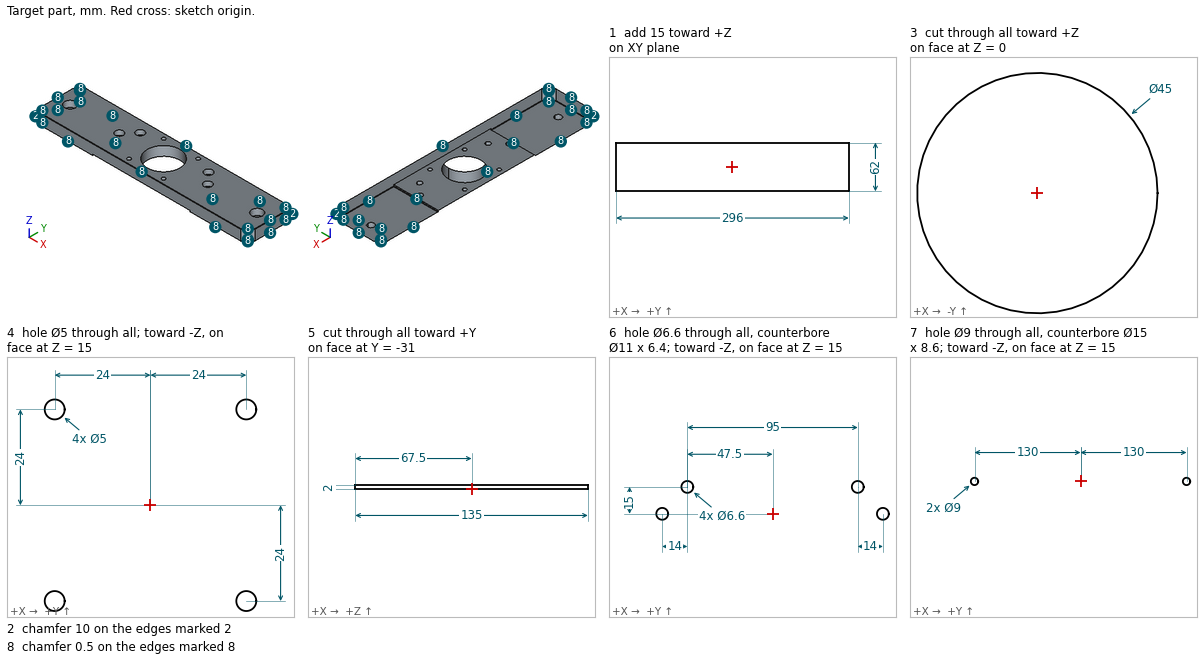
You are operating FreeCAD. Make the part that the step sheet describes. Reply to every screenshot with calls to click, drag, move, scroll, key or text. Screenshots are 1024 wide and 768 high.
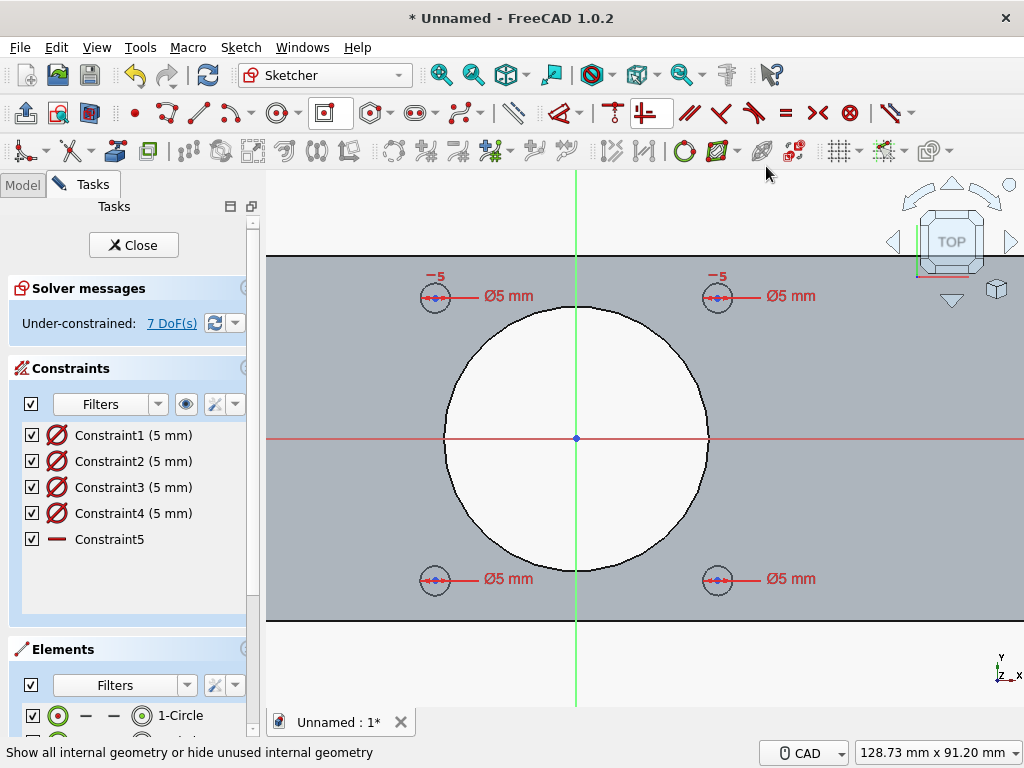
click(718, 298)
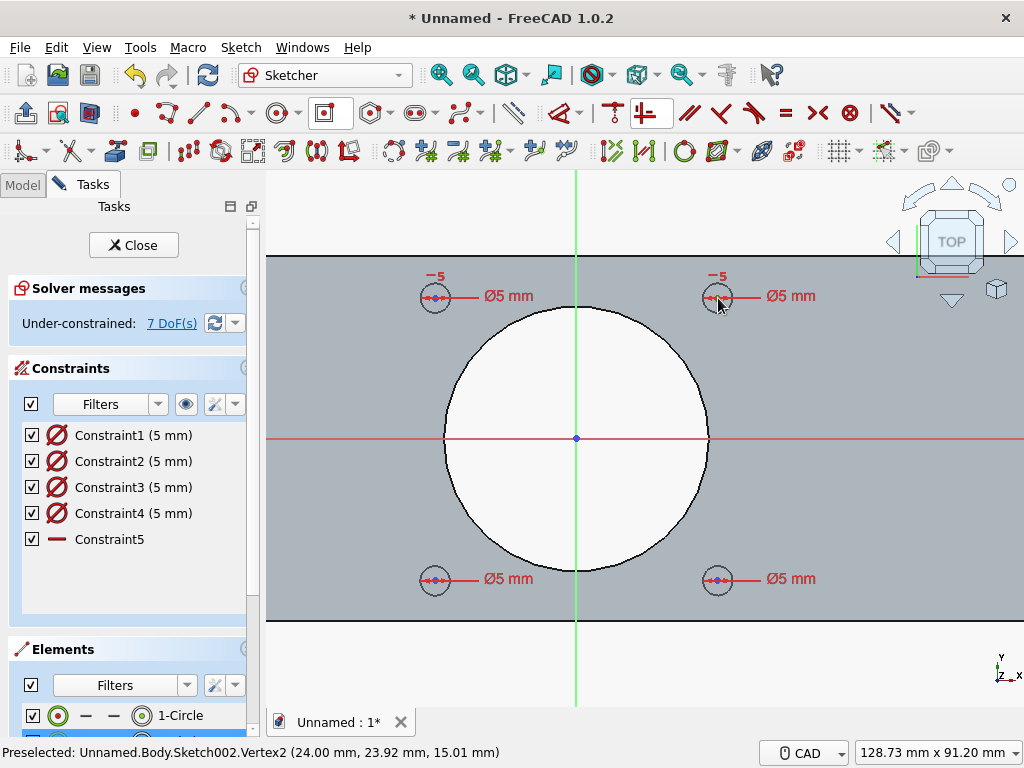
click(718, 581)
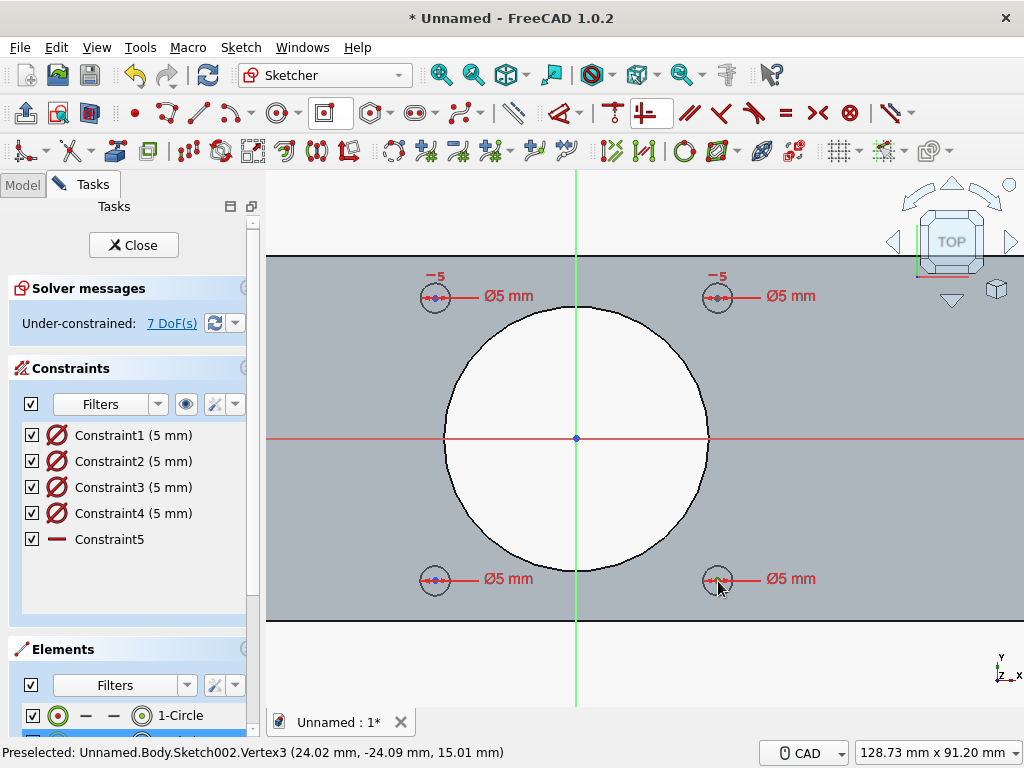
click(668, 114)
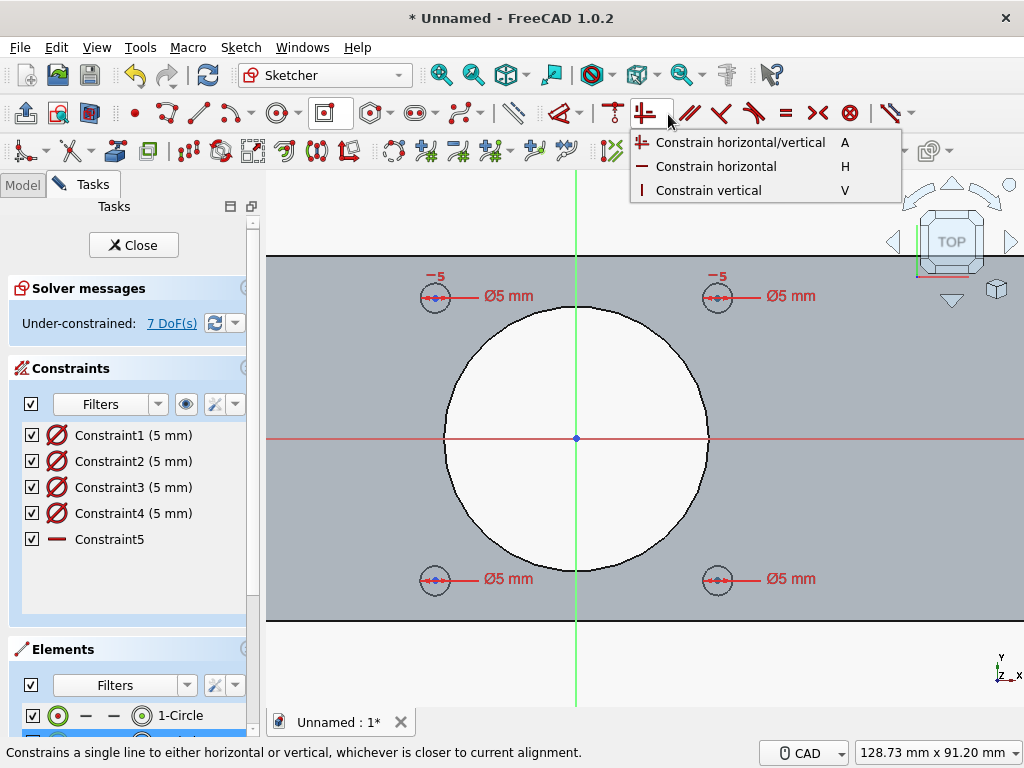
click(766, 190)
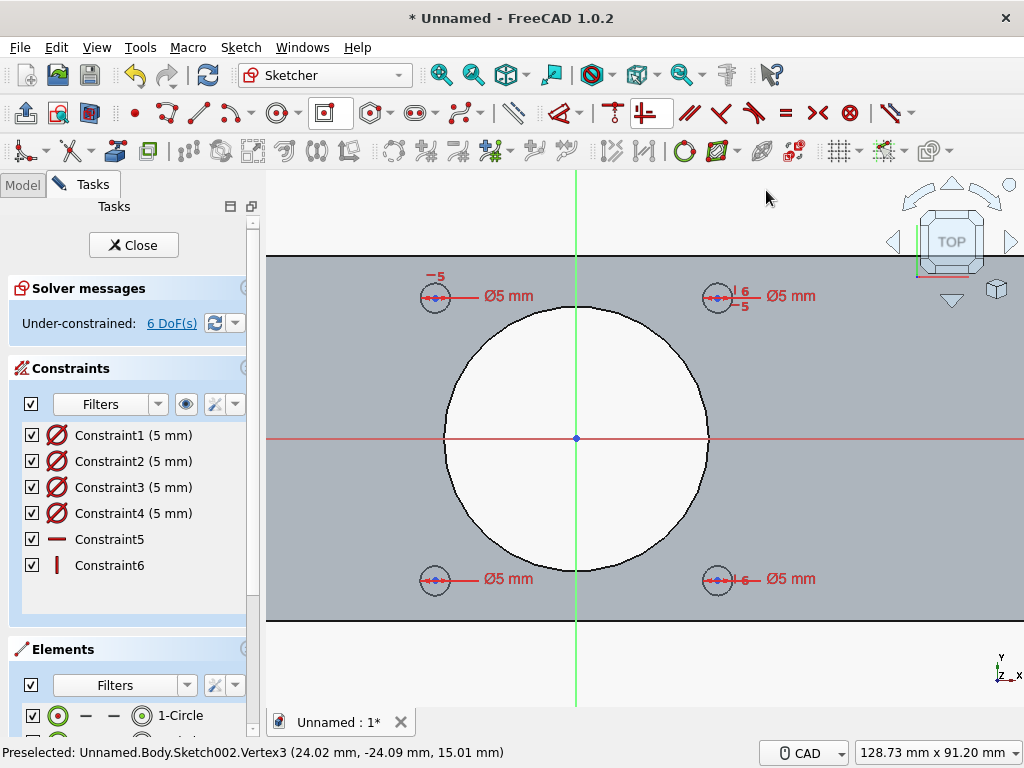
click(435, 298)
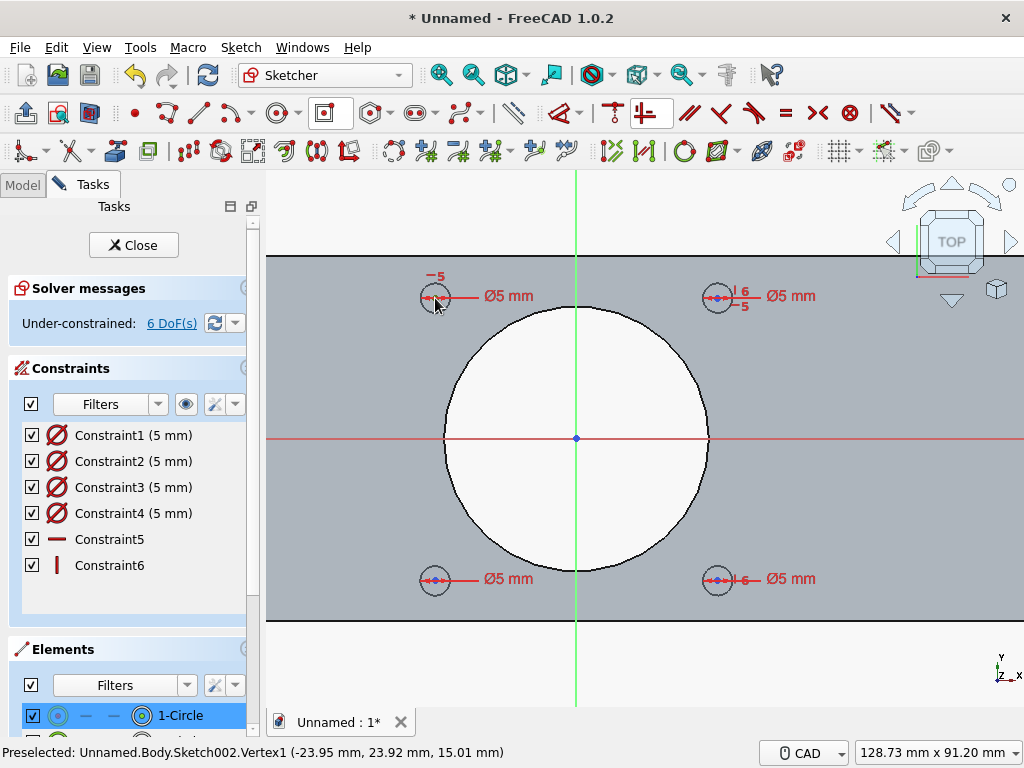
click(435, 581)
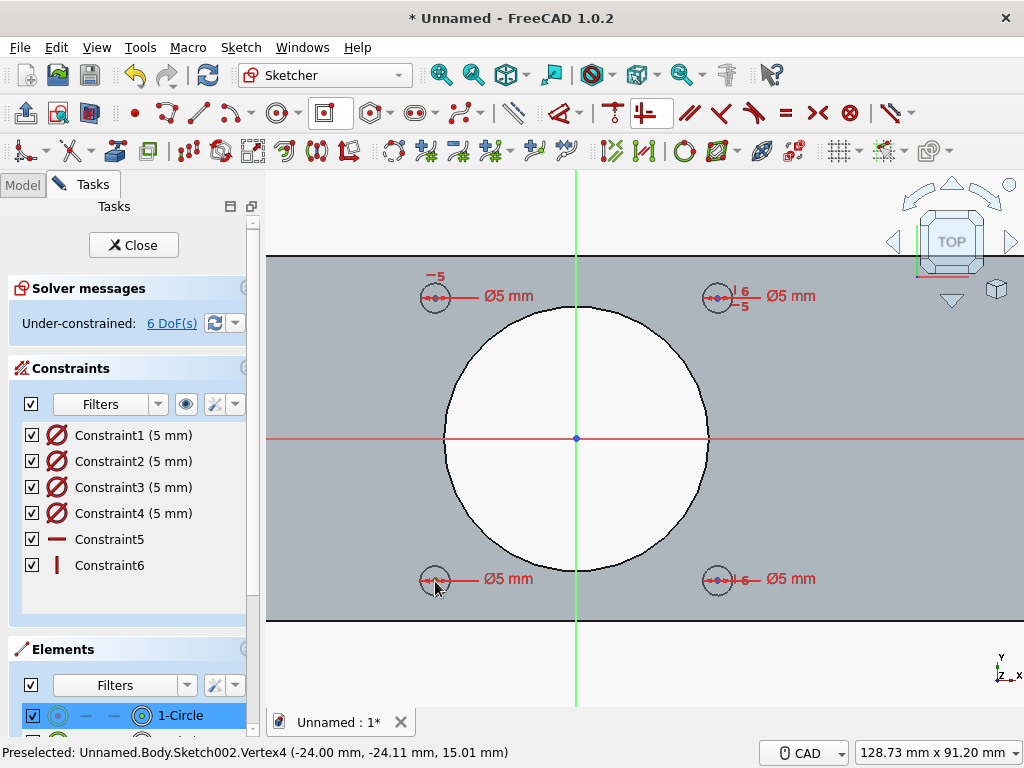
click(668, 114)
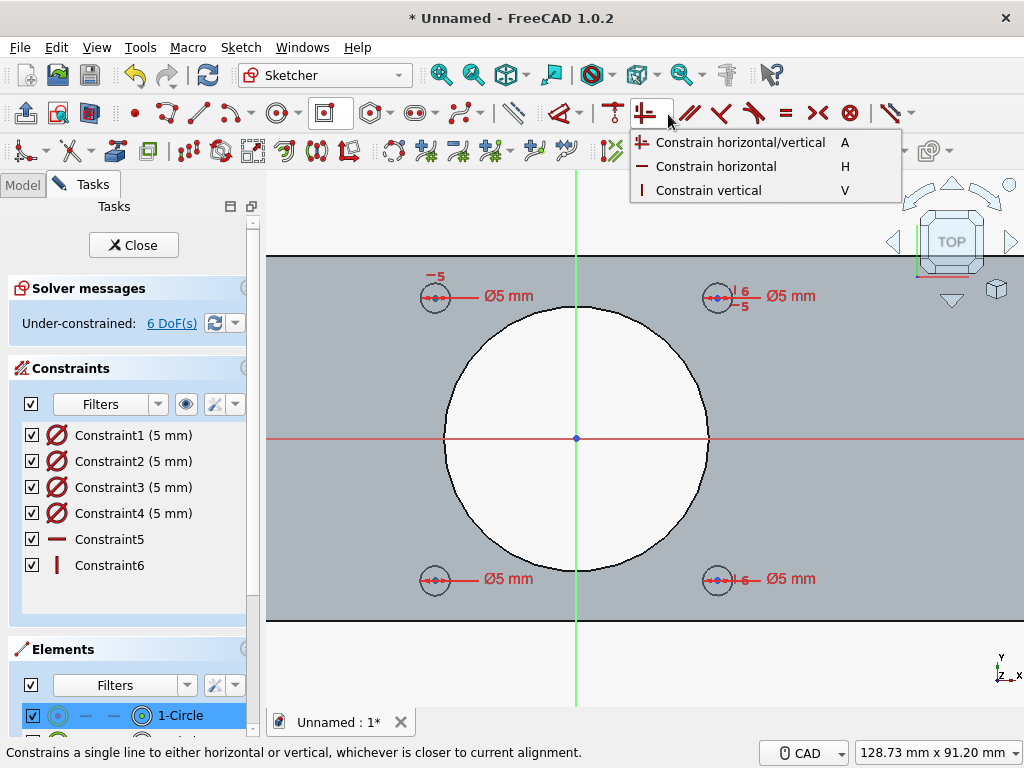
click(766, 190)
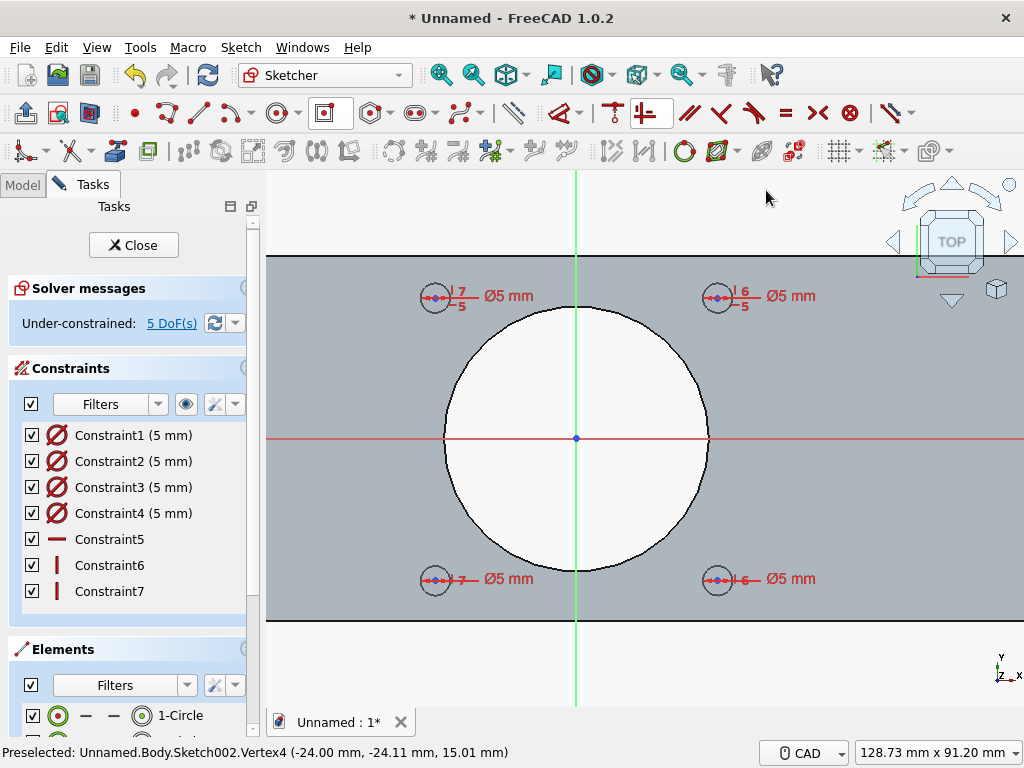
click(718, 581)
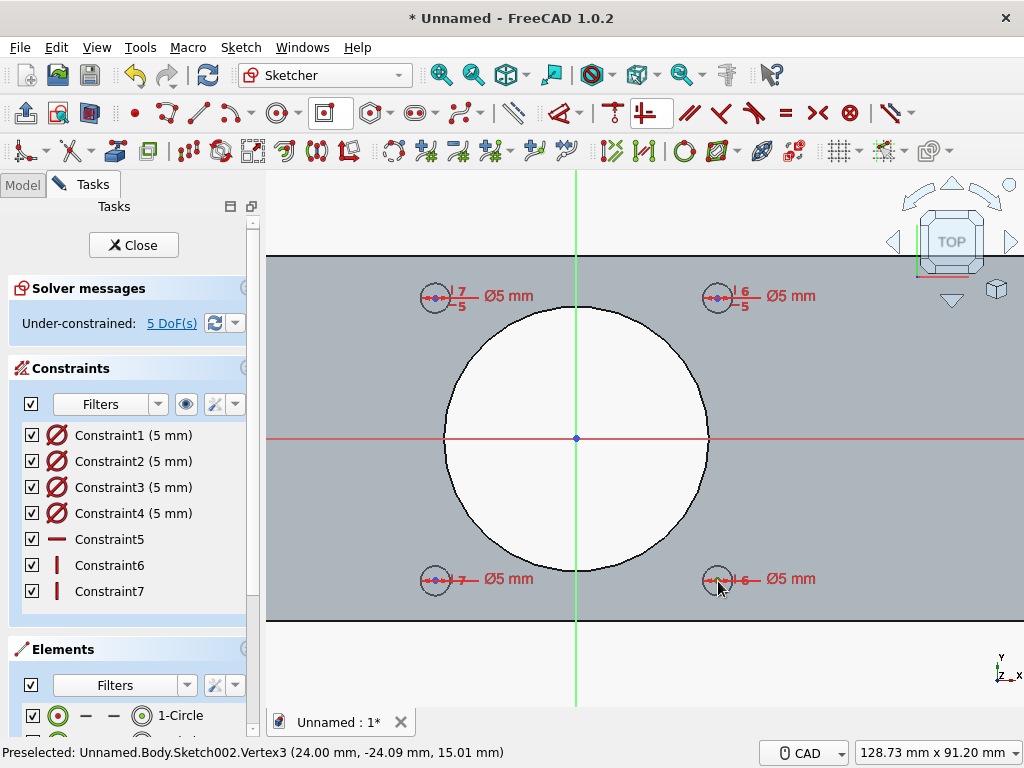
click(435, 581)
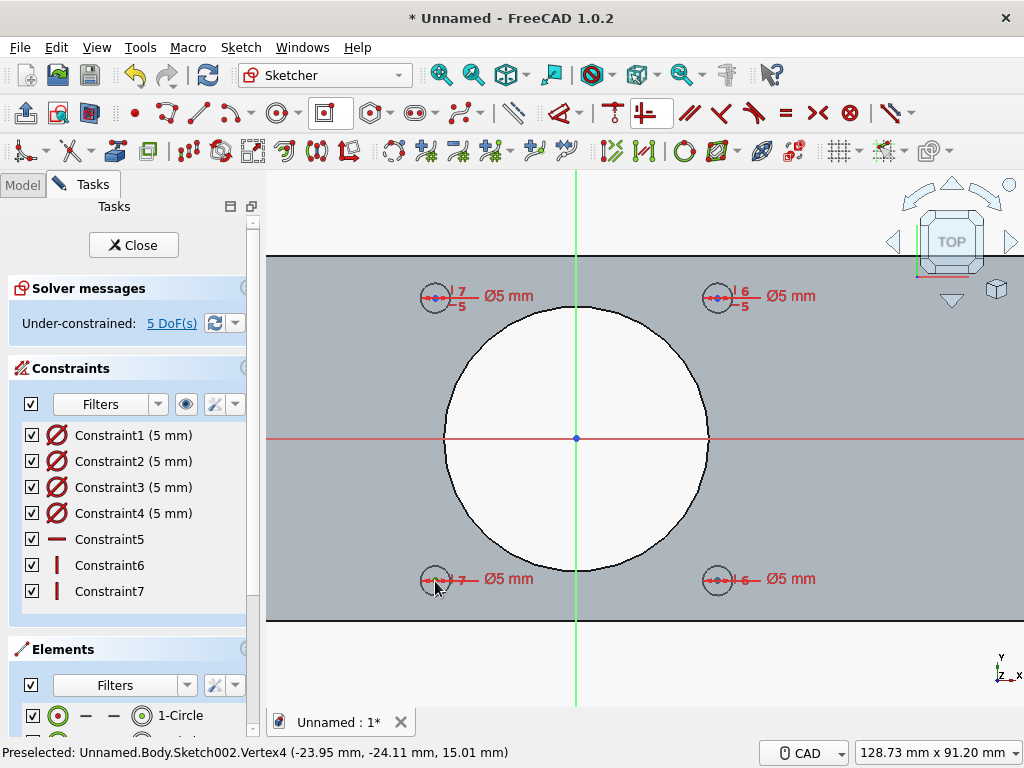
key(h)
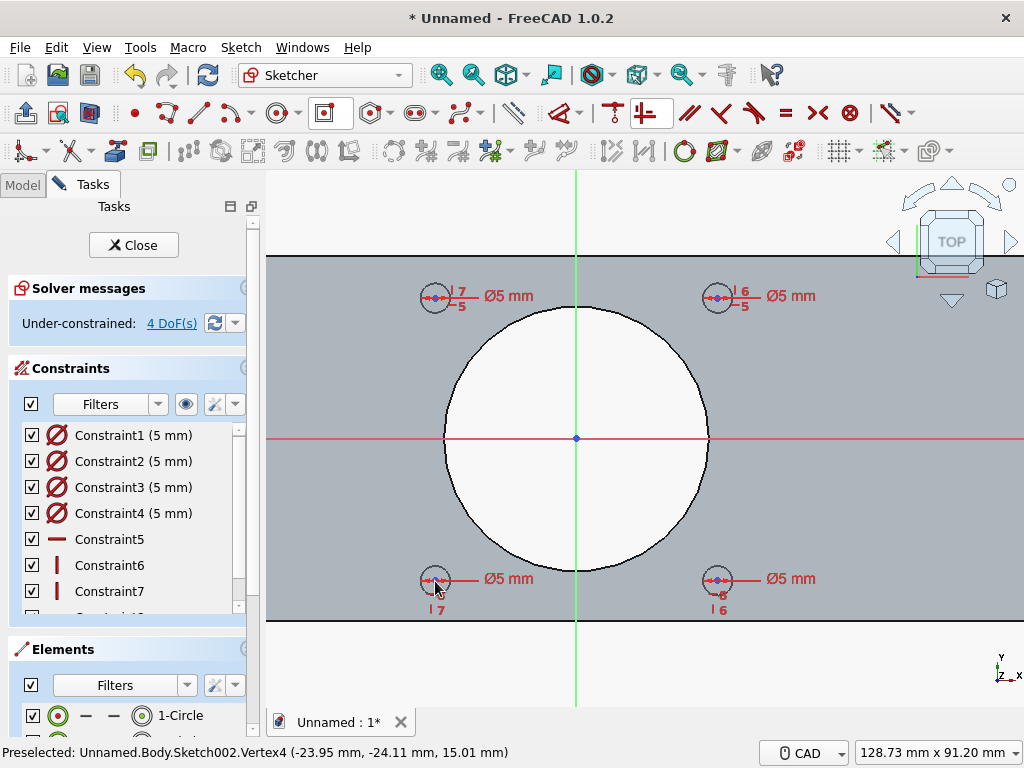
click(560, 114)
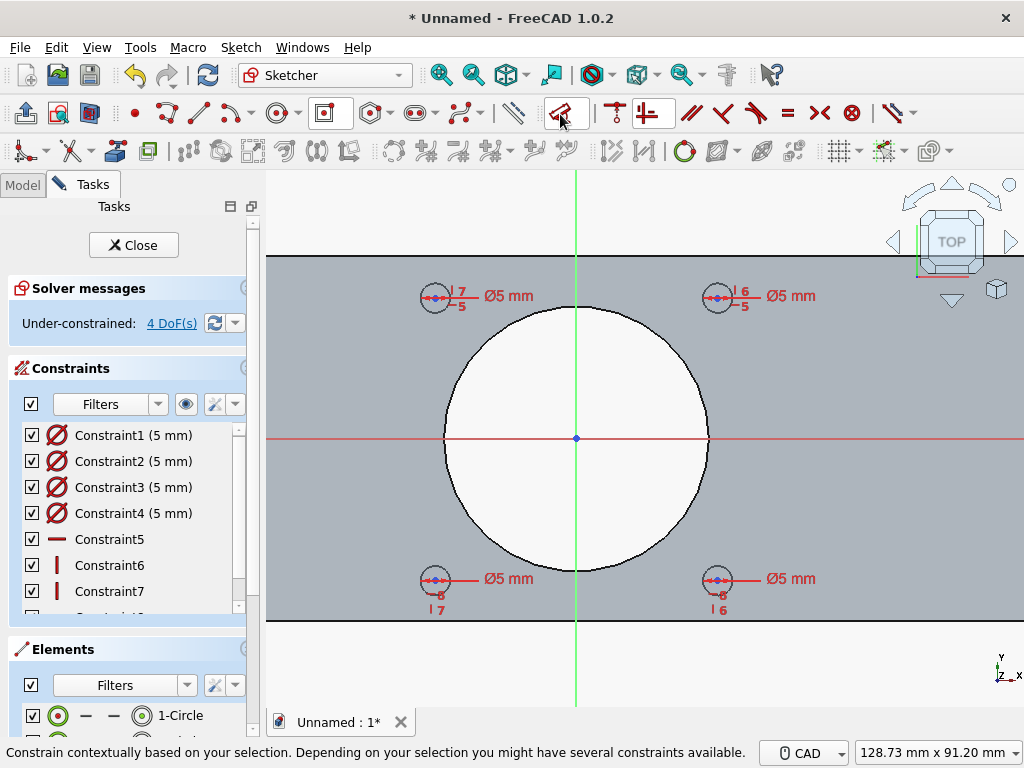
click(435, 298)
click(506, 264)